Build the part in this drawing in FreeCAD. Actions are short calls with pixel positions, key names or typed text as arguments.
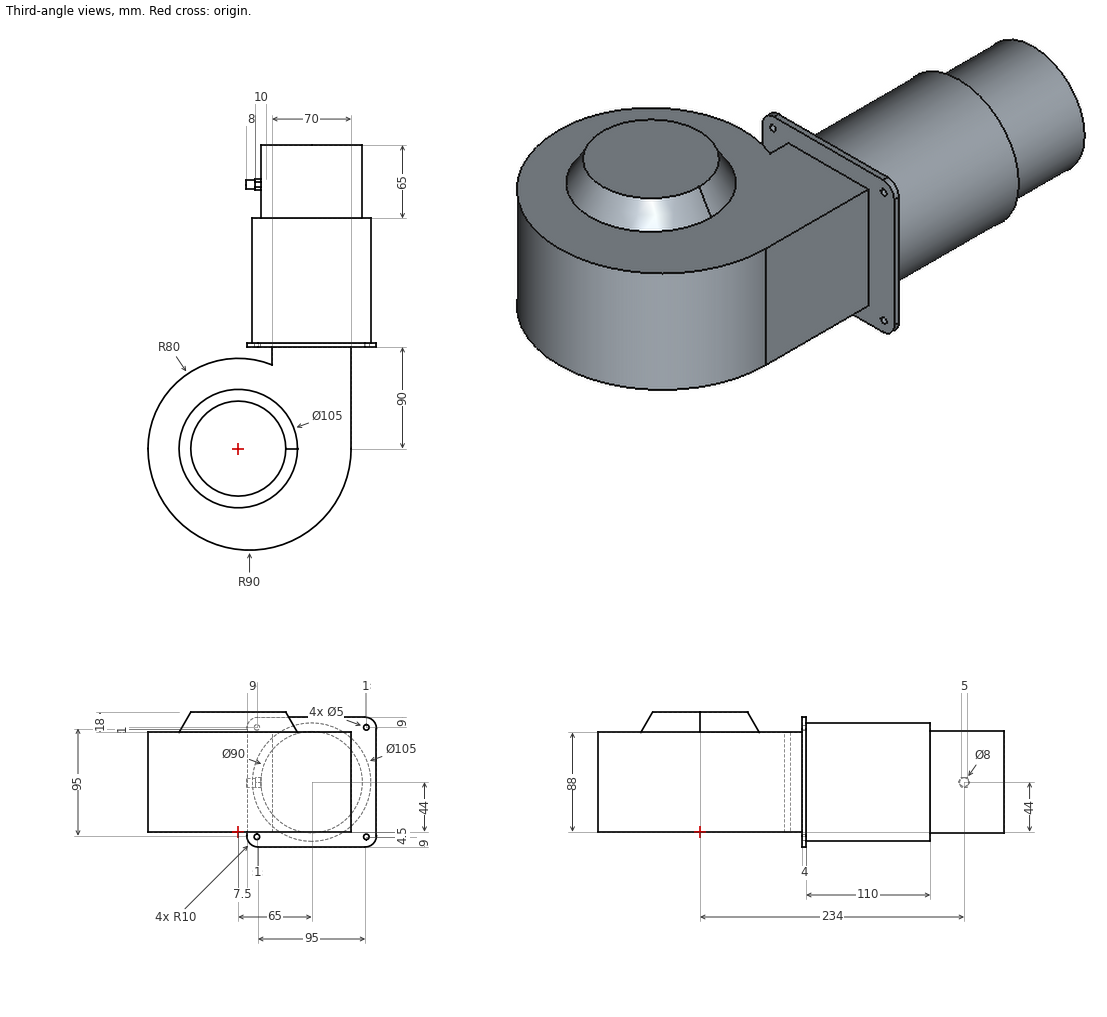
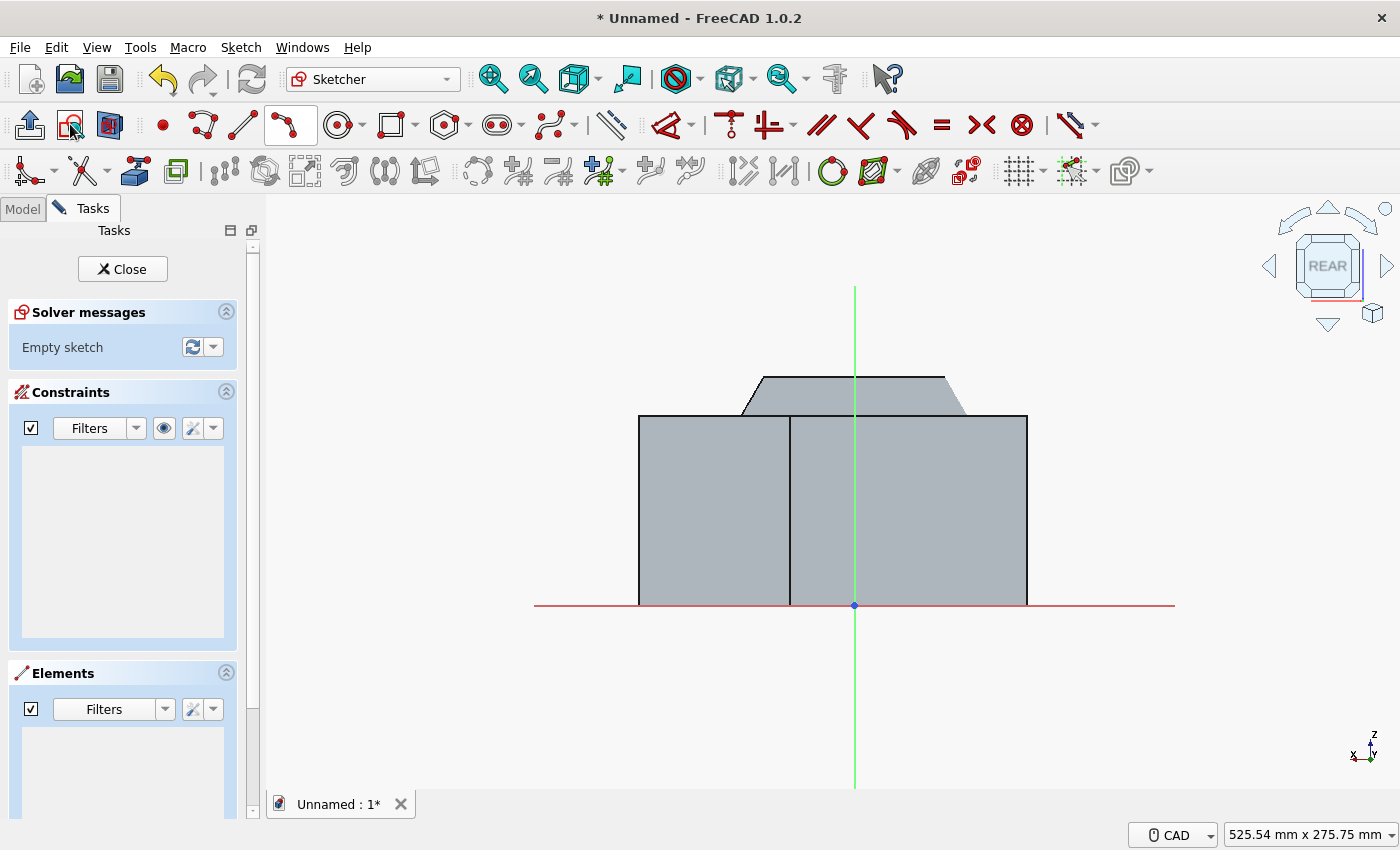
scroll(637, 550, up, 2)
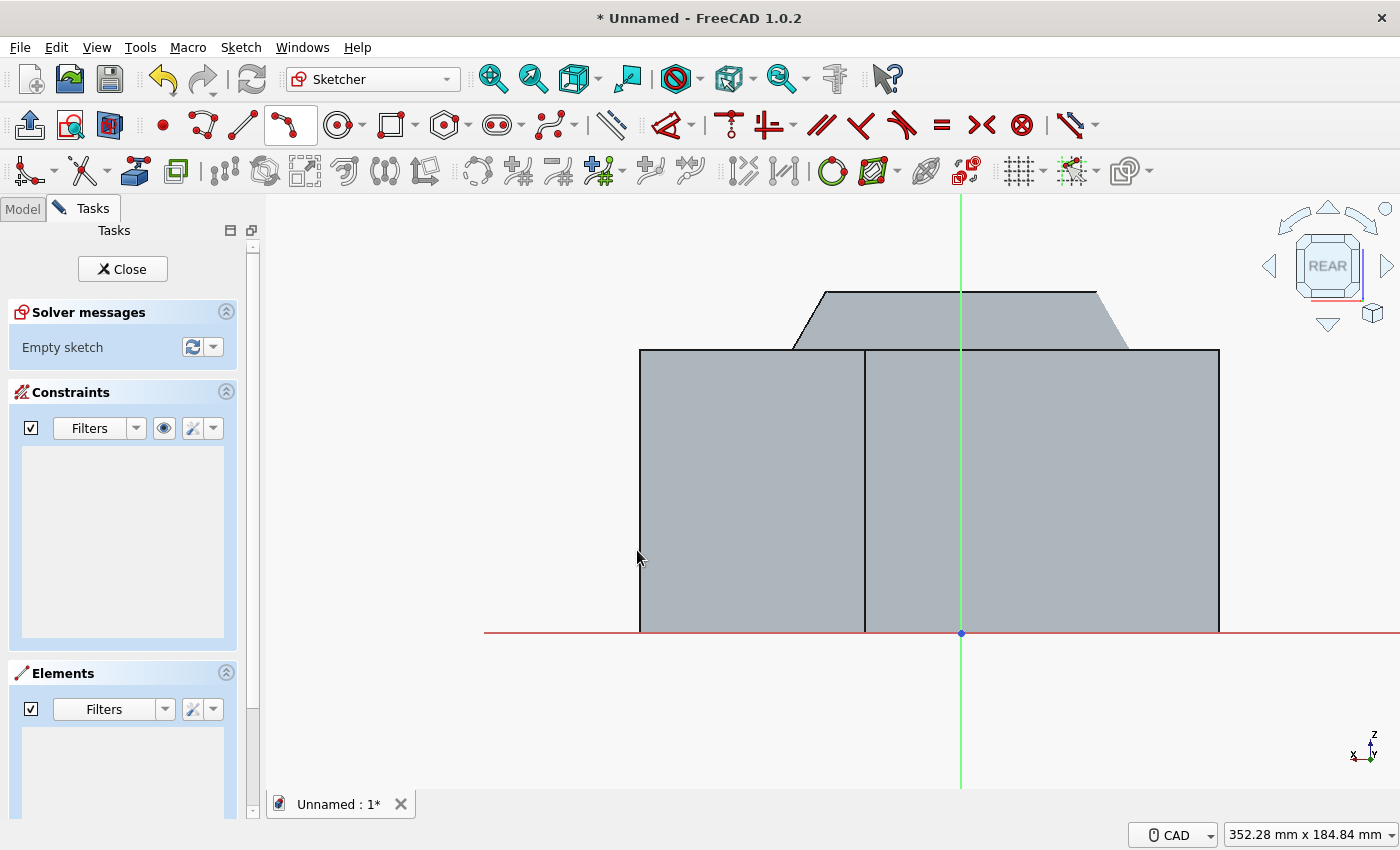
click(244, 126)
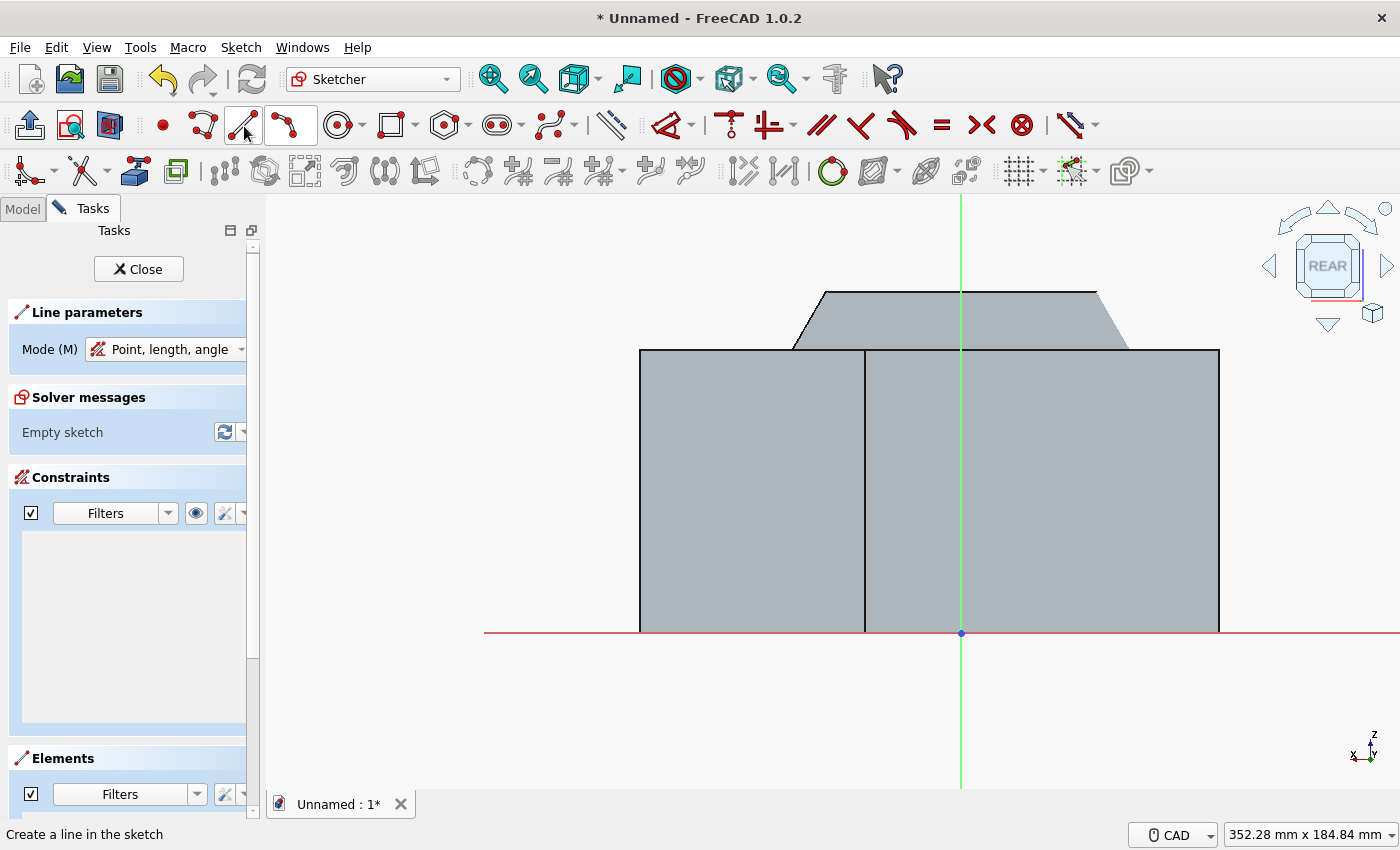
click(599, 676)
click(905, 676)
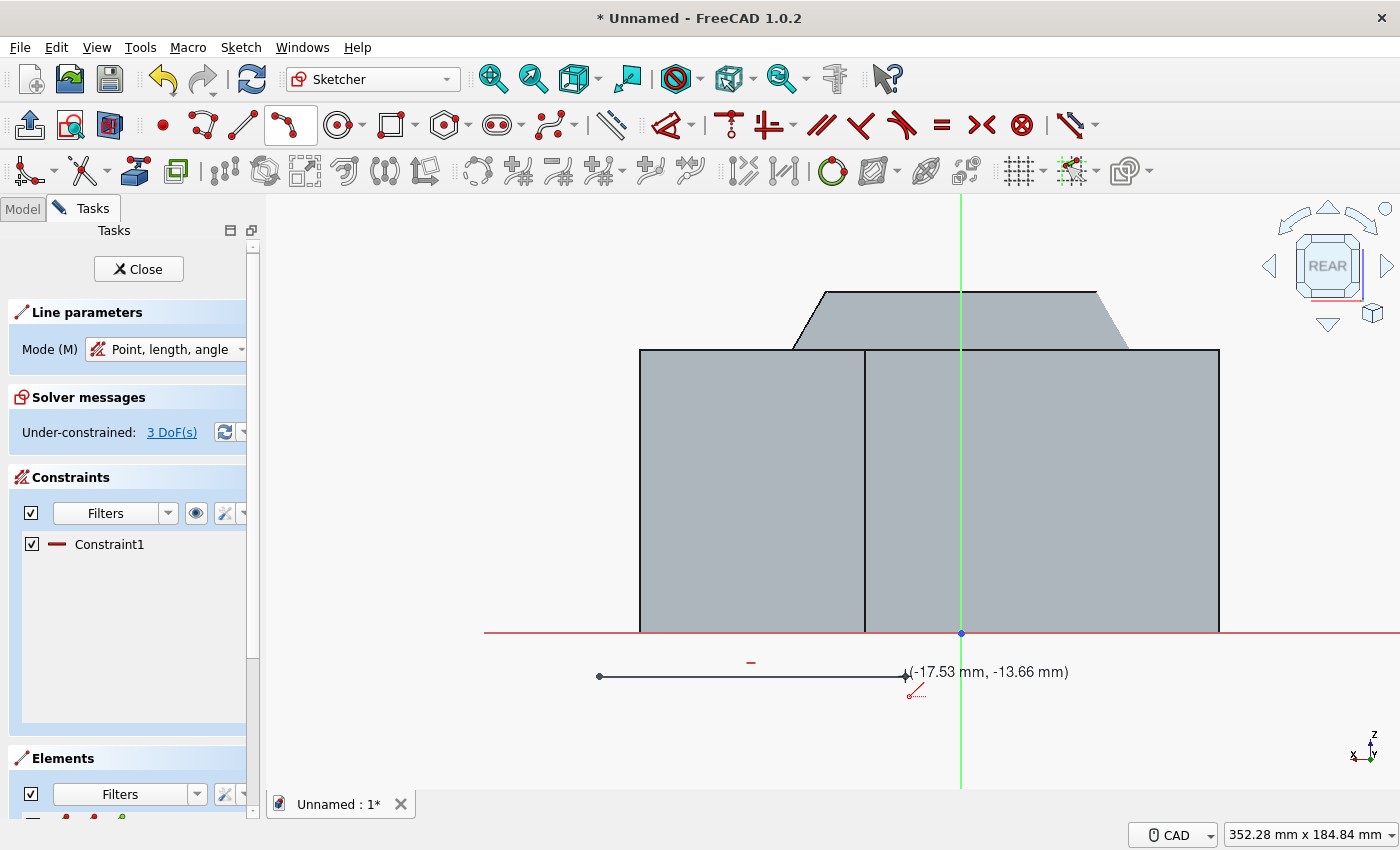
scroll(937, 644, up, 2)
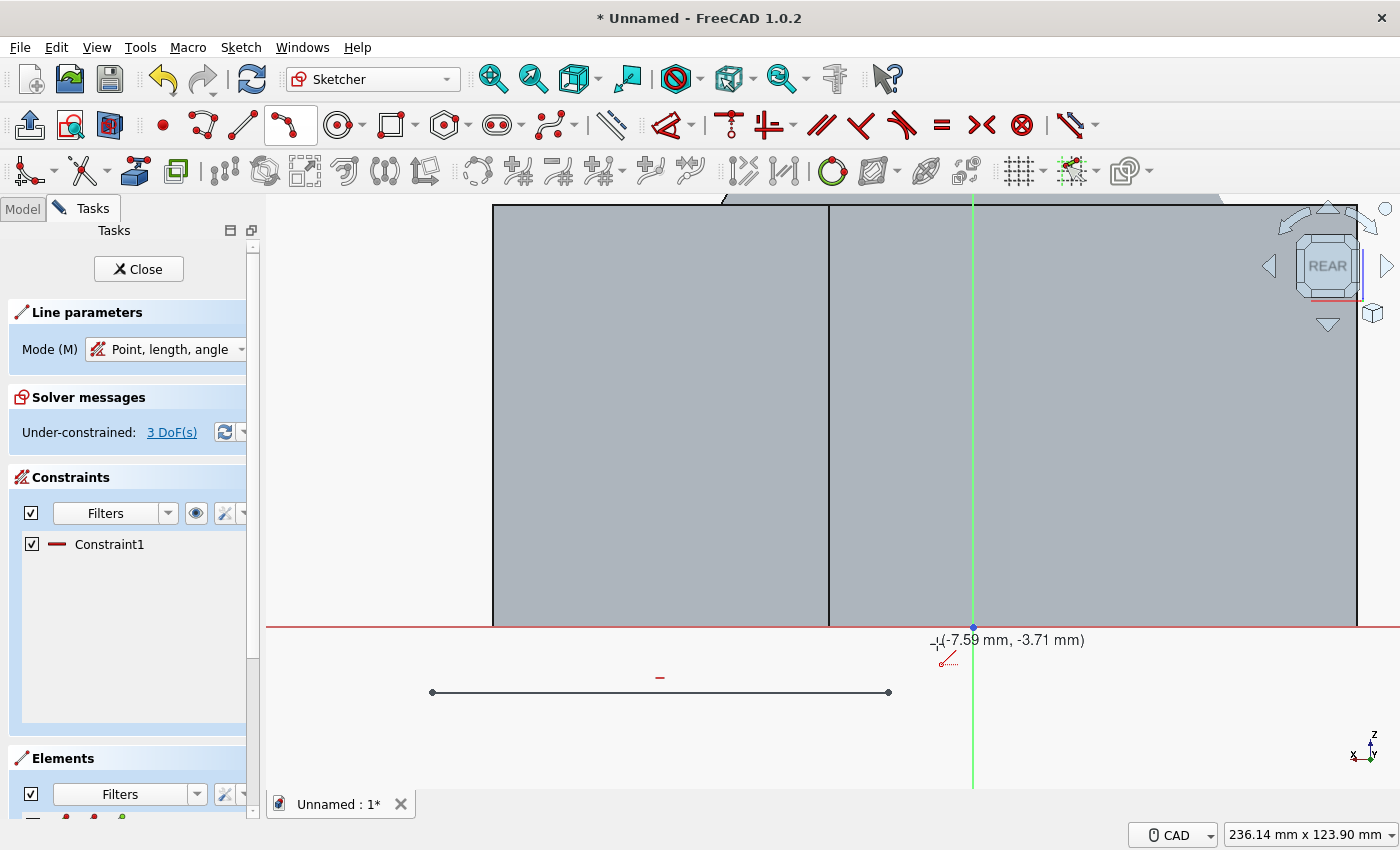
click(937, 644)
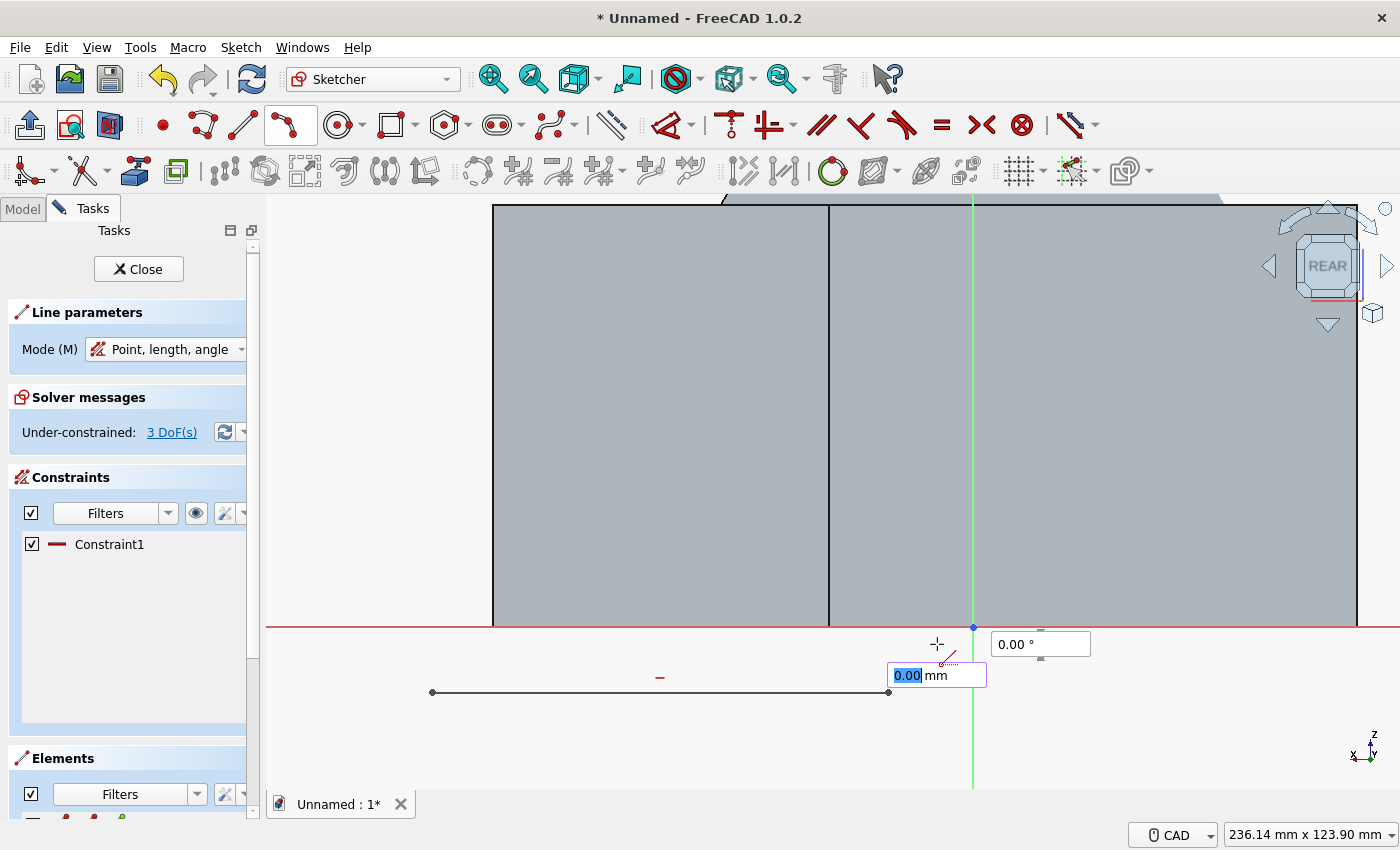
scroll(938, 645, down, 2)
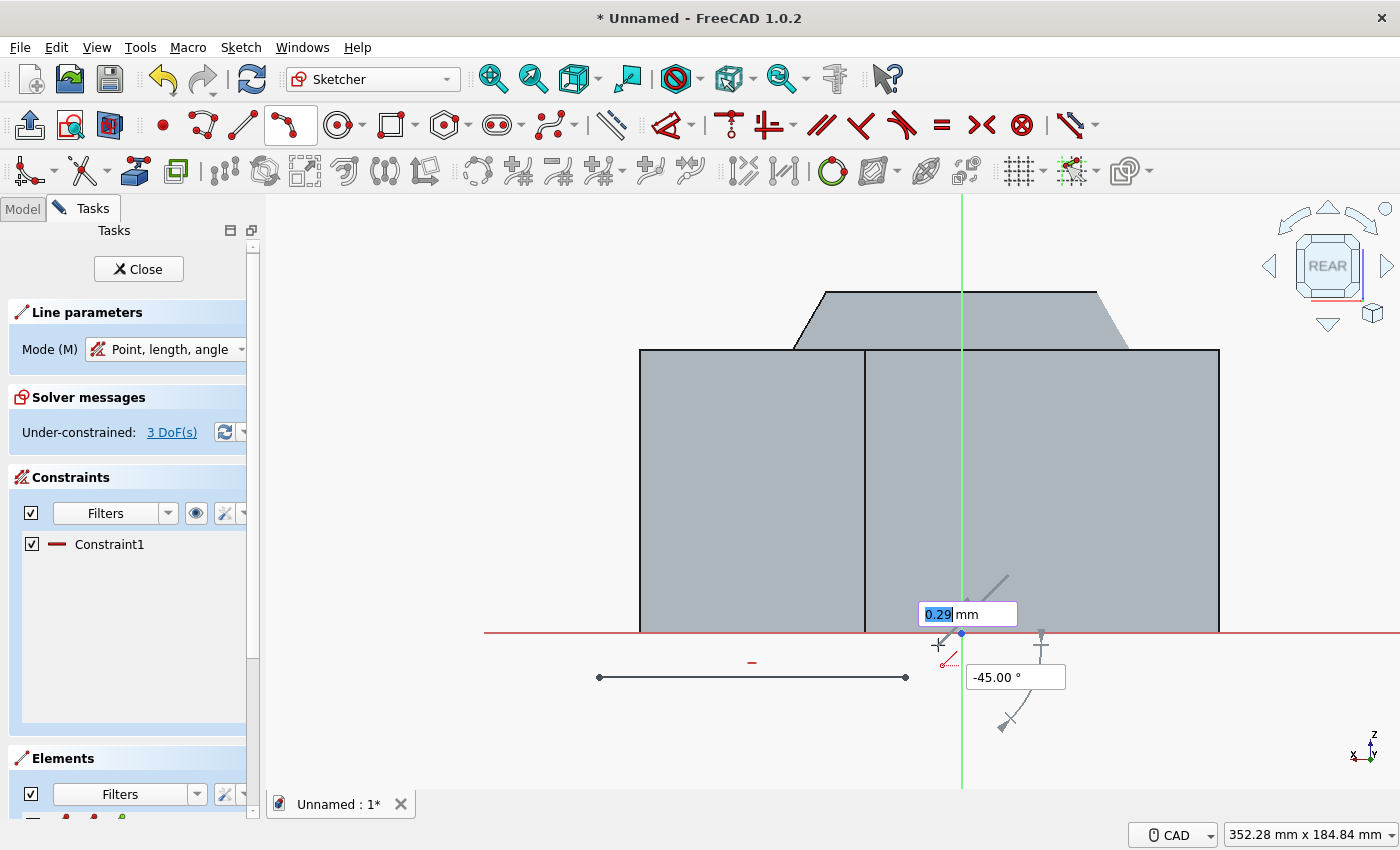
click(938, 339)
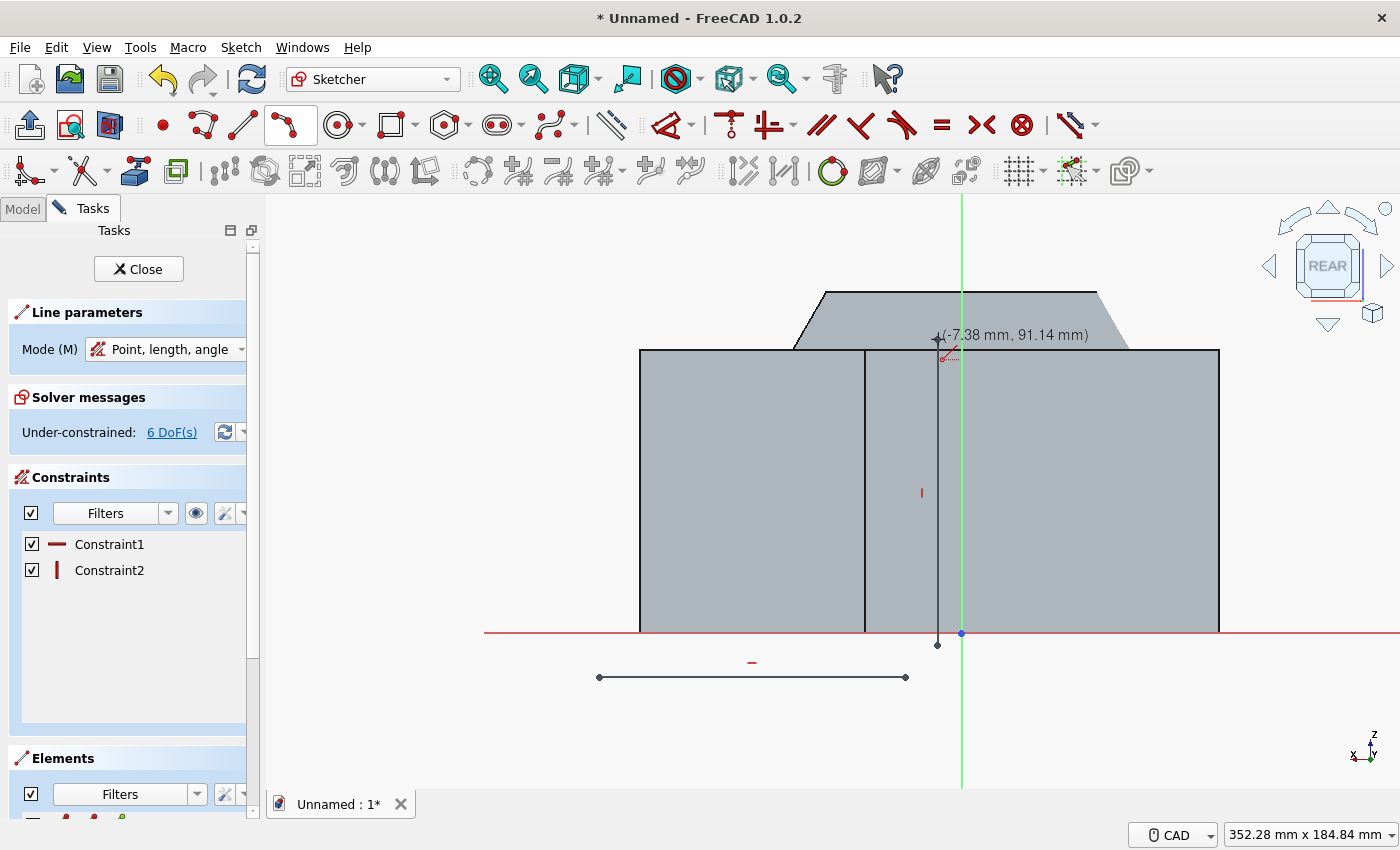
click(905, 307)
click(600, 307)